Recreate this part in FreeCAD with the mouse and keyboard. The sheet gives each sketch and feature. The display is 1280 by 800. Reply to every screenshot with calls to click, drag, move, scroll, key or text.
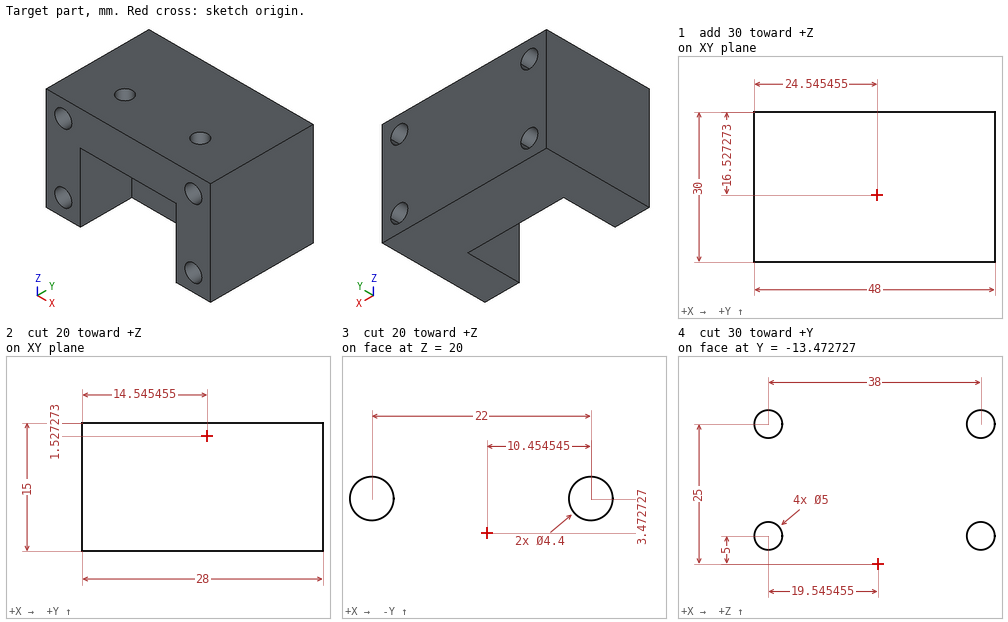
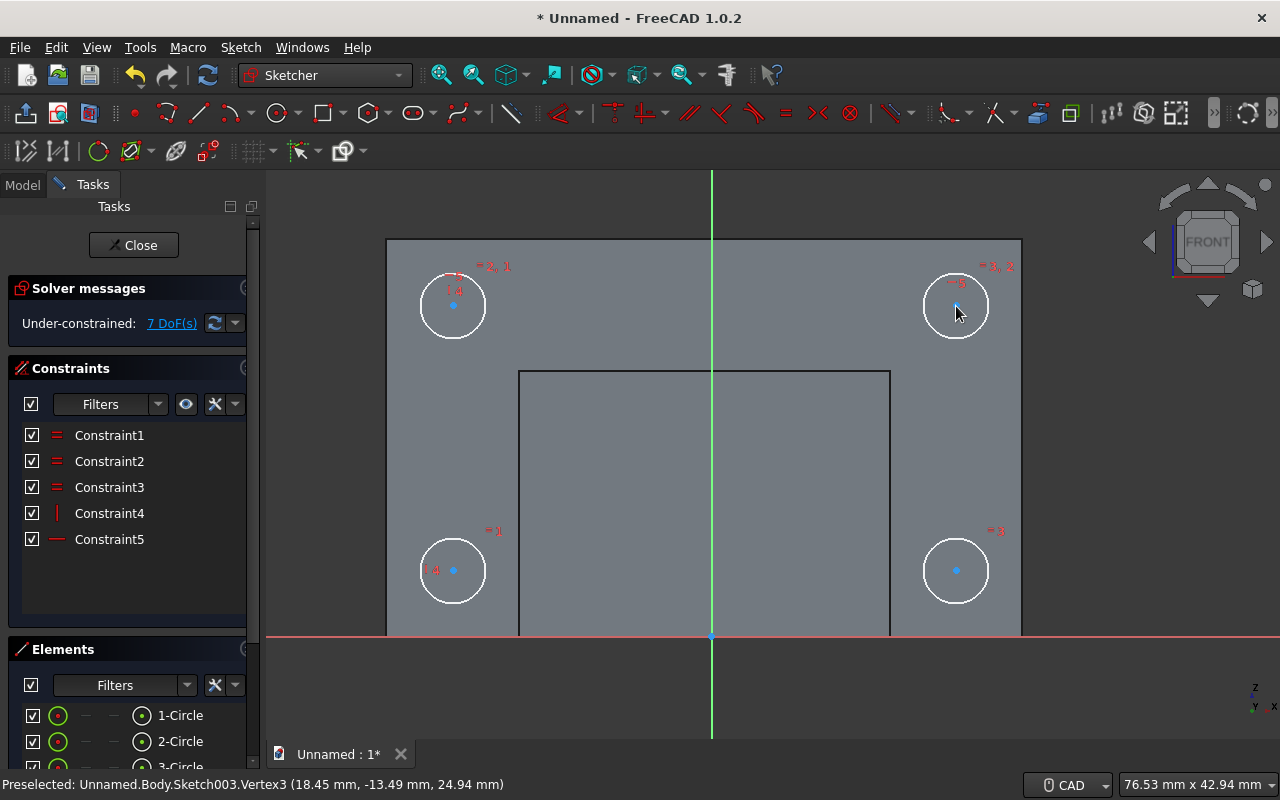
click(956, 306)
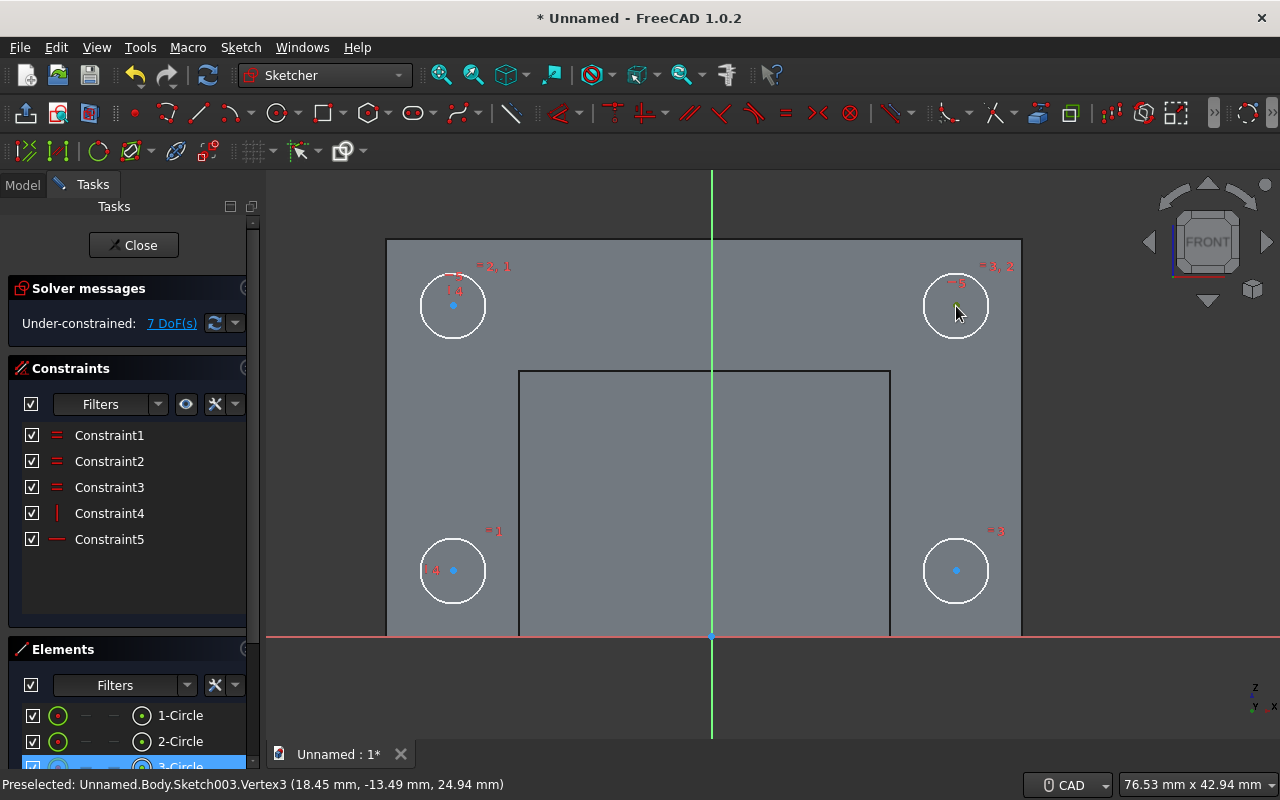
click(956, 571)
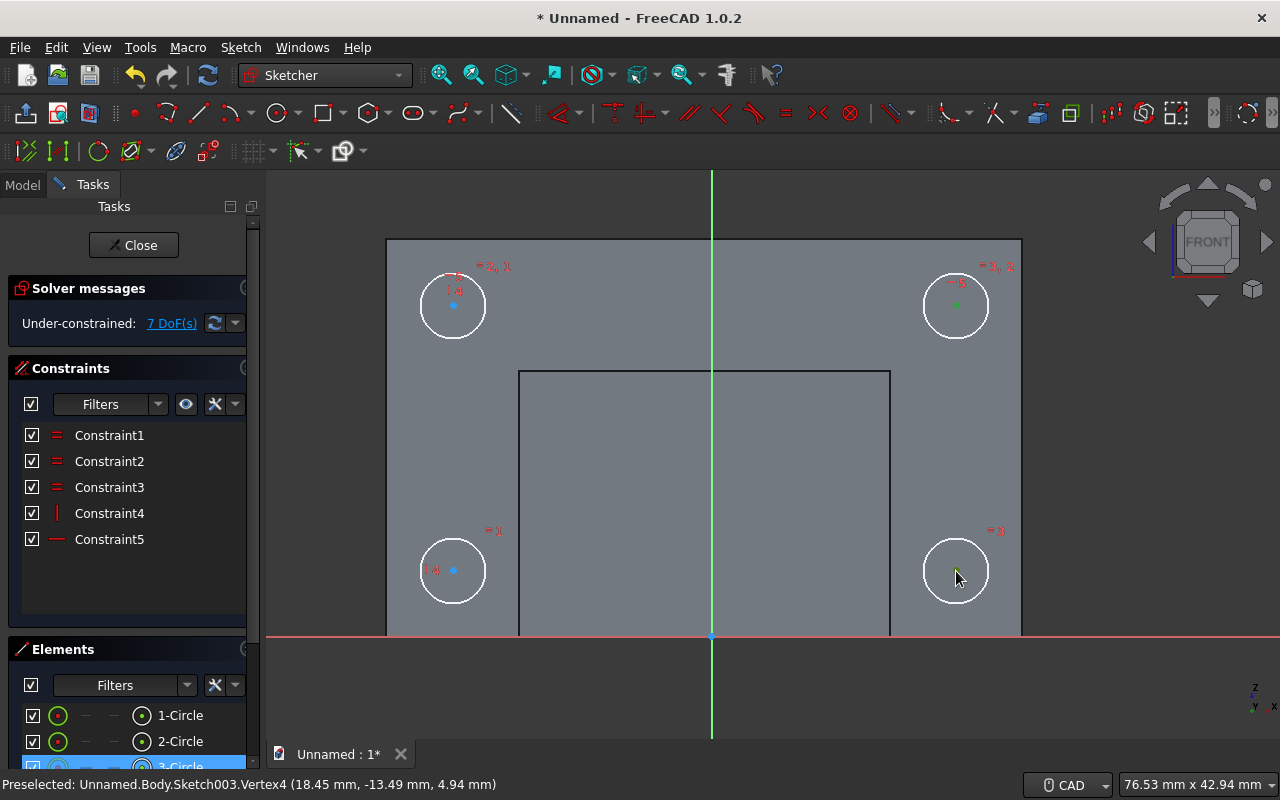
click(668, 114)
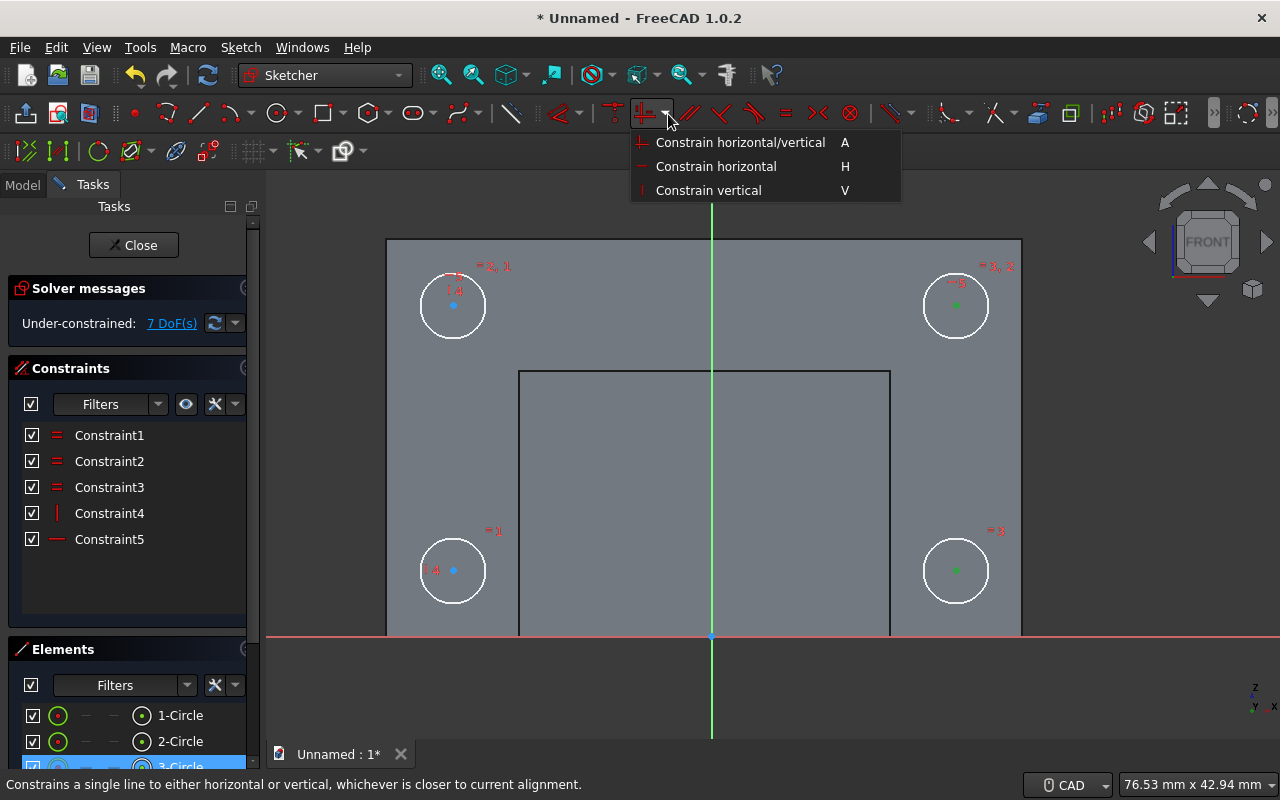
click(766, 190)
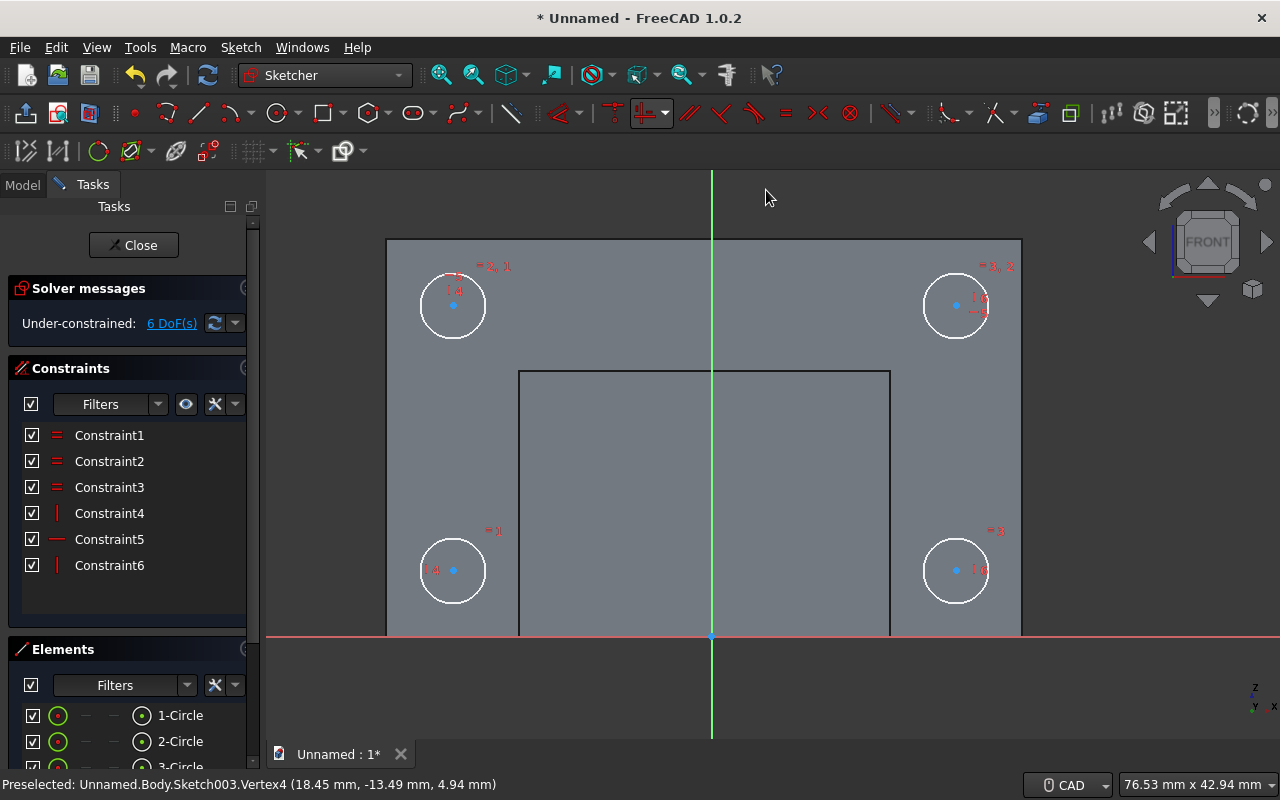
click(453, 571)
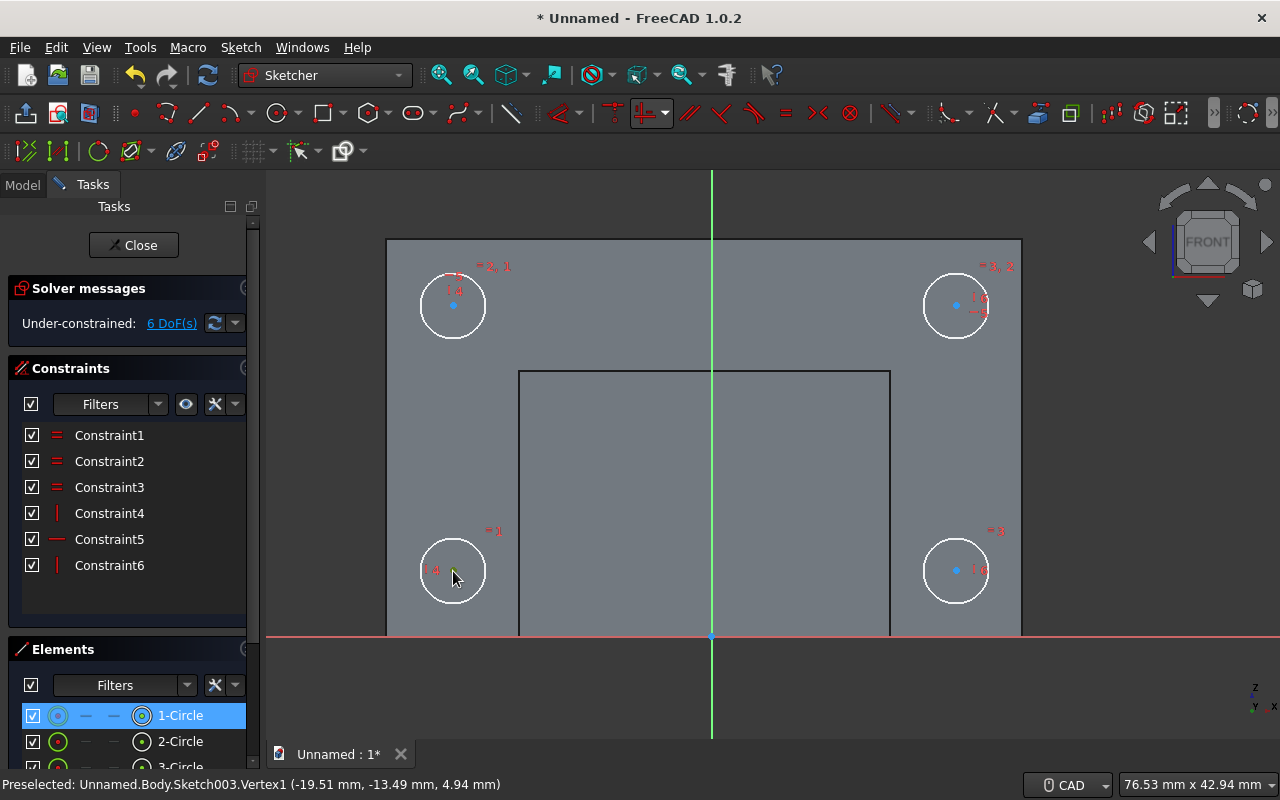
click(956, 571)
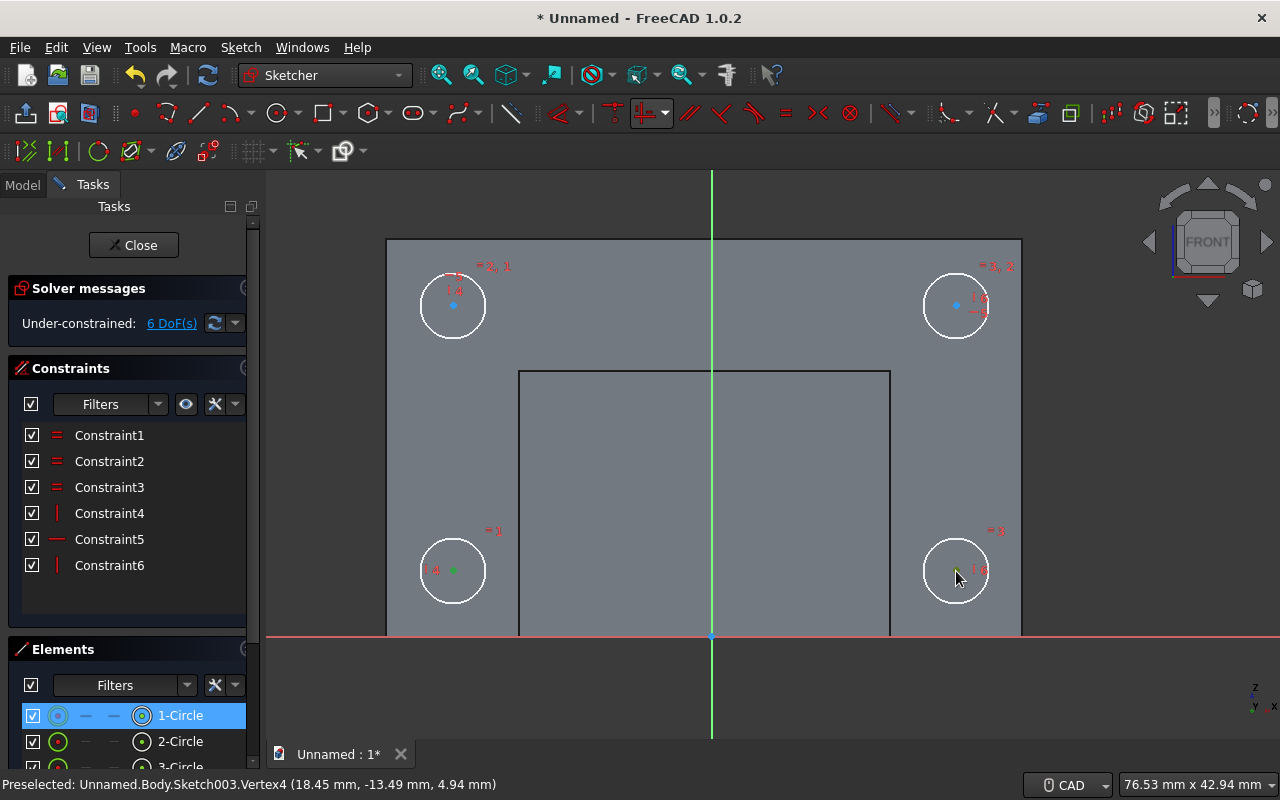
click(668, 114)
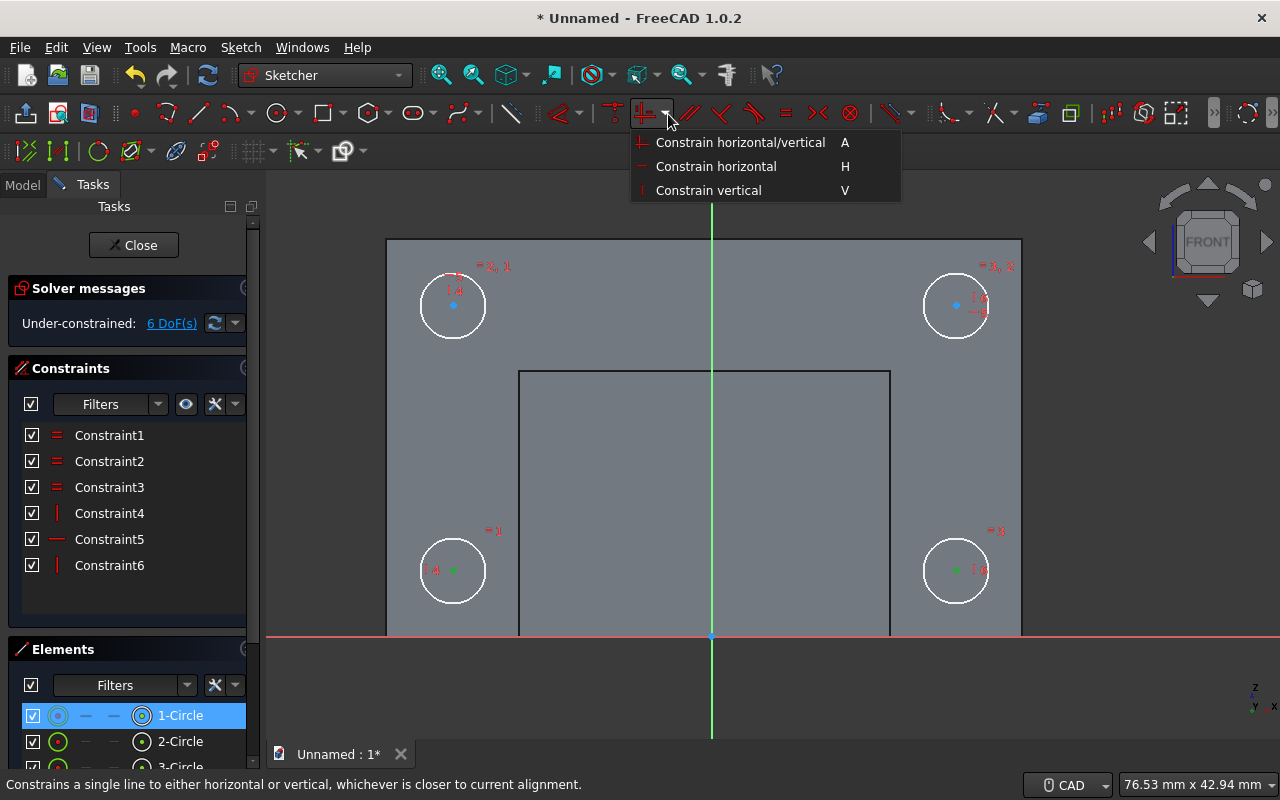
click(766, 166)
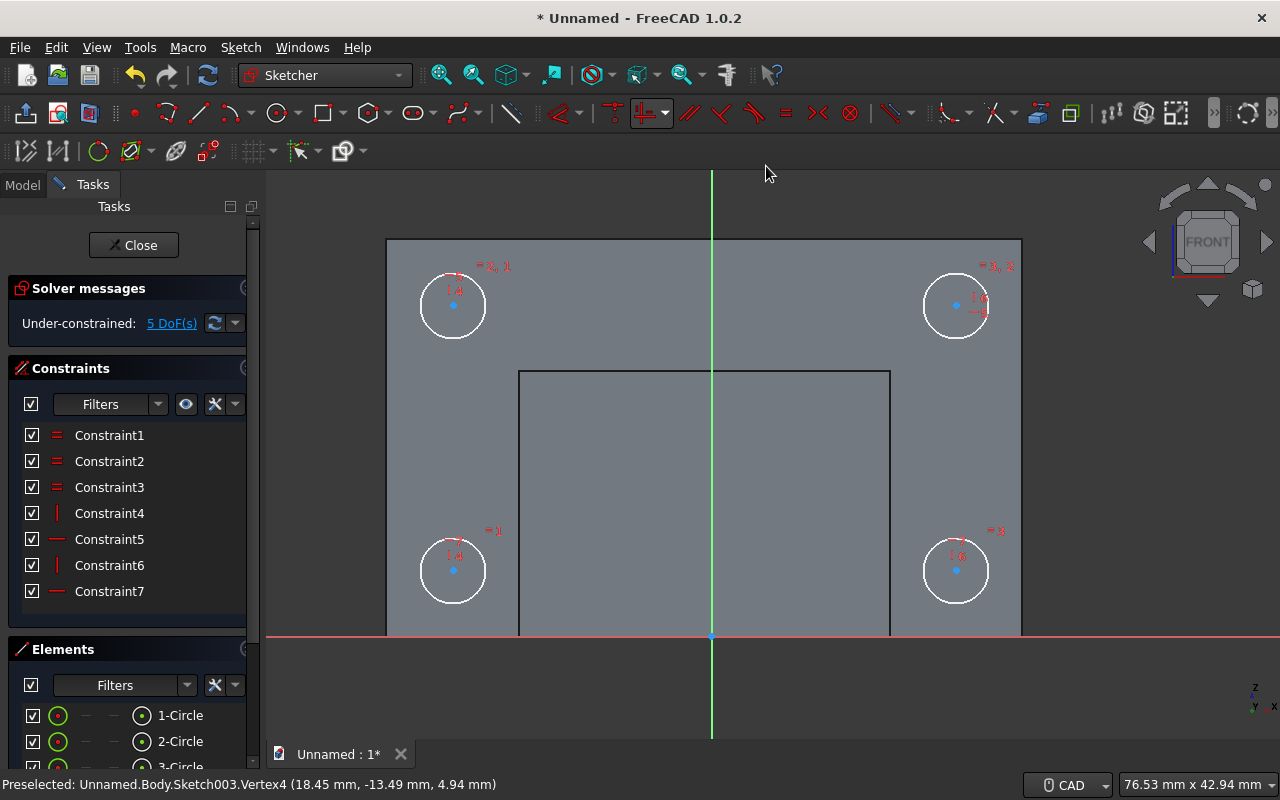
click(558, 114)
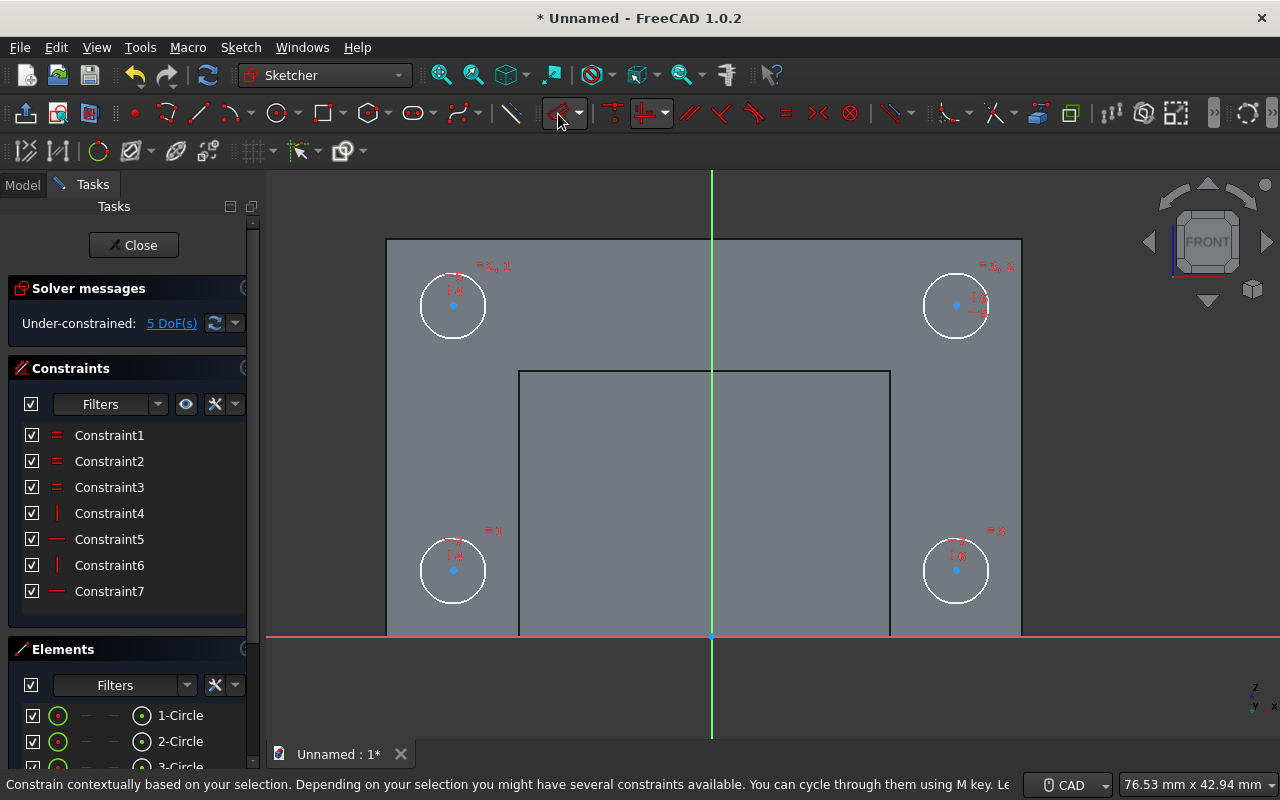
click(476, 548)
click(499, 525)